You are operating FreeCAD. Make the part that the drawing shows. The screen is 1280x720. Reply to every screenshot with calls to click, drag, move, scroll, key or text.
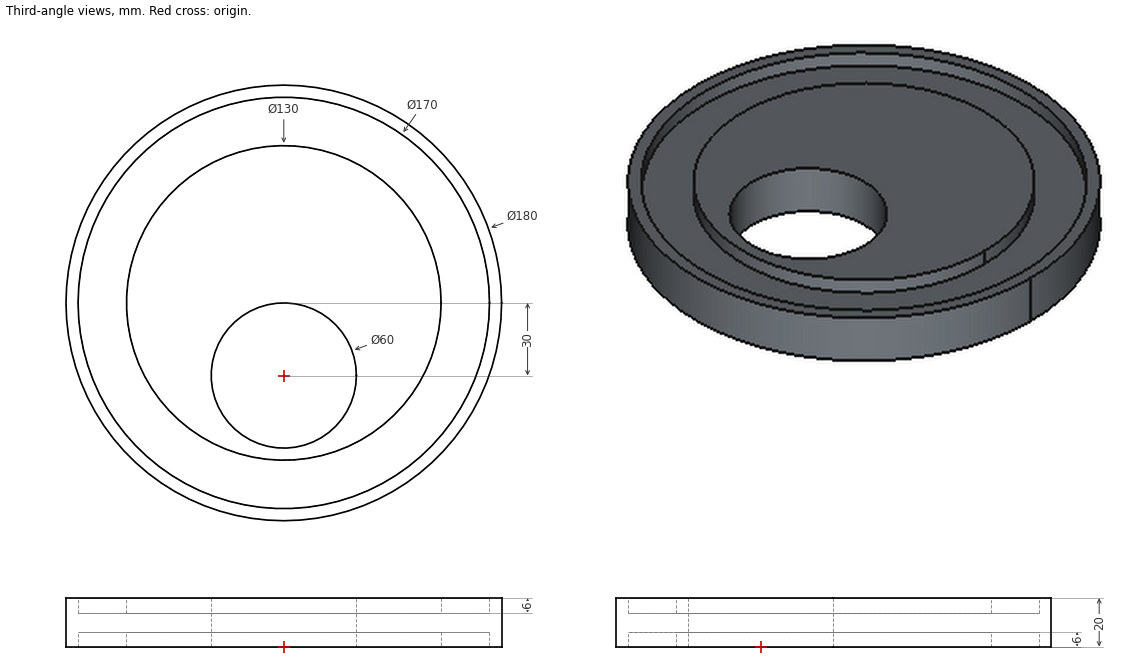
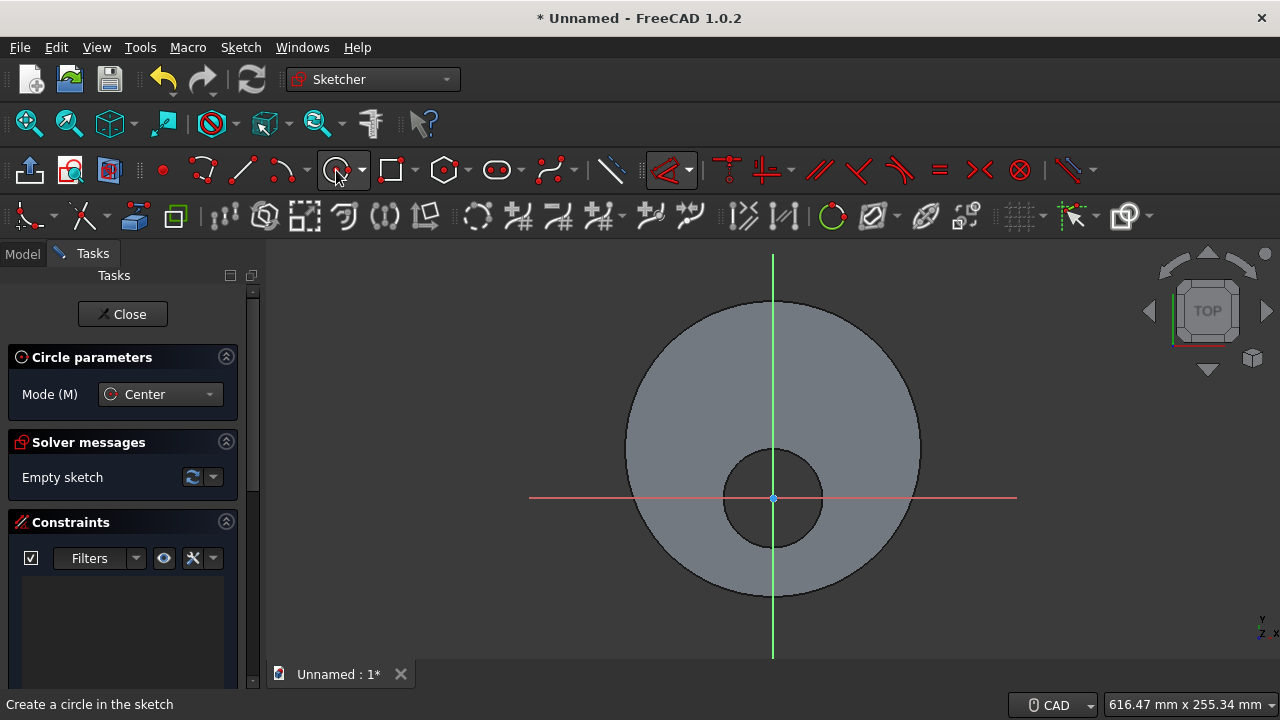
click(773, 449)
move(872, 350)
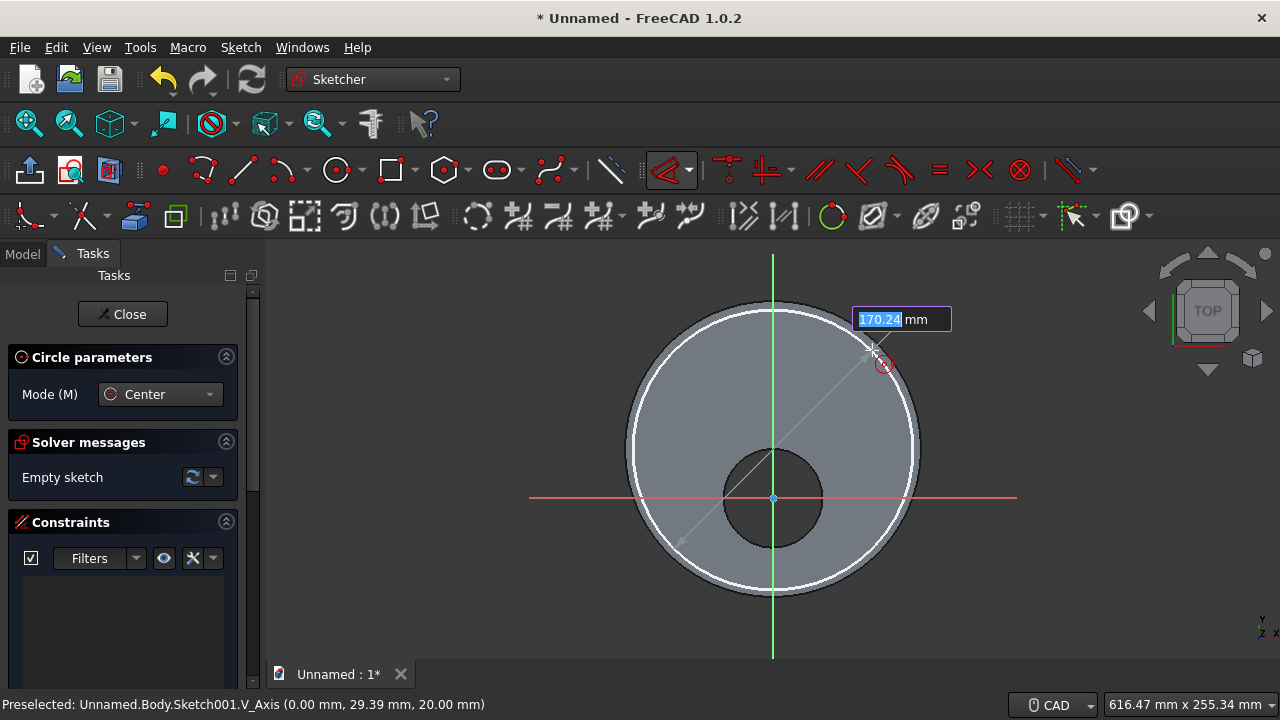
text(170)
key(Return)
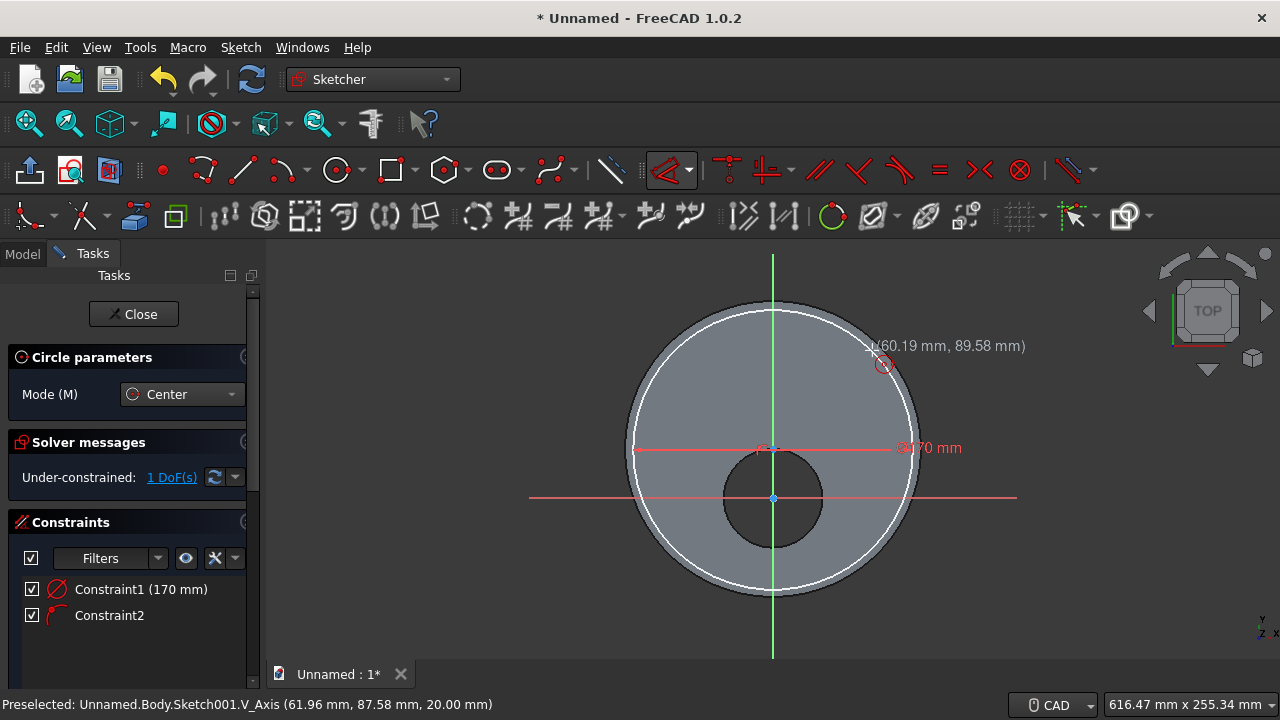
click(773, 450)
move(849, 373)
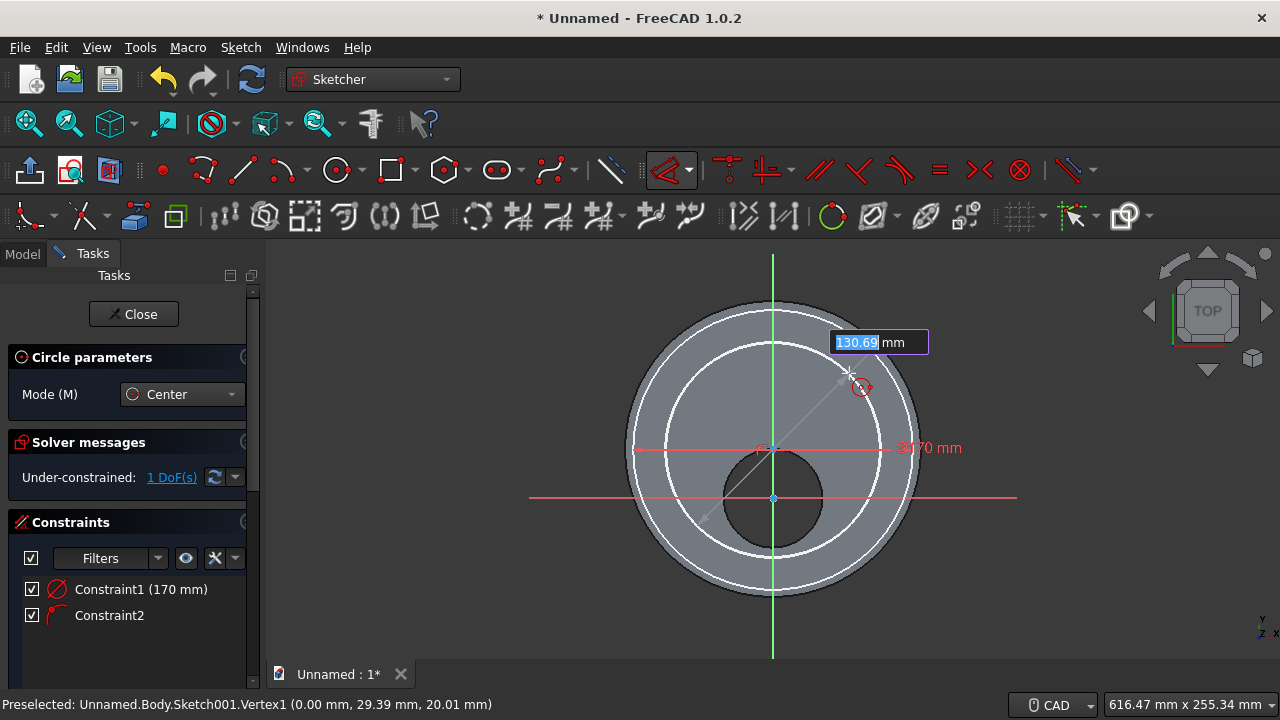
text(130)
key(Return)
key(Escape)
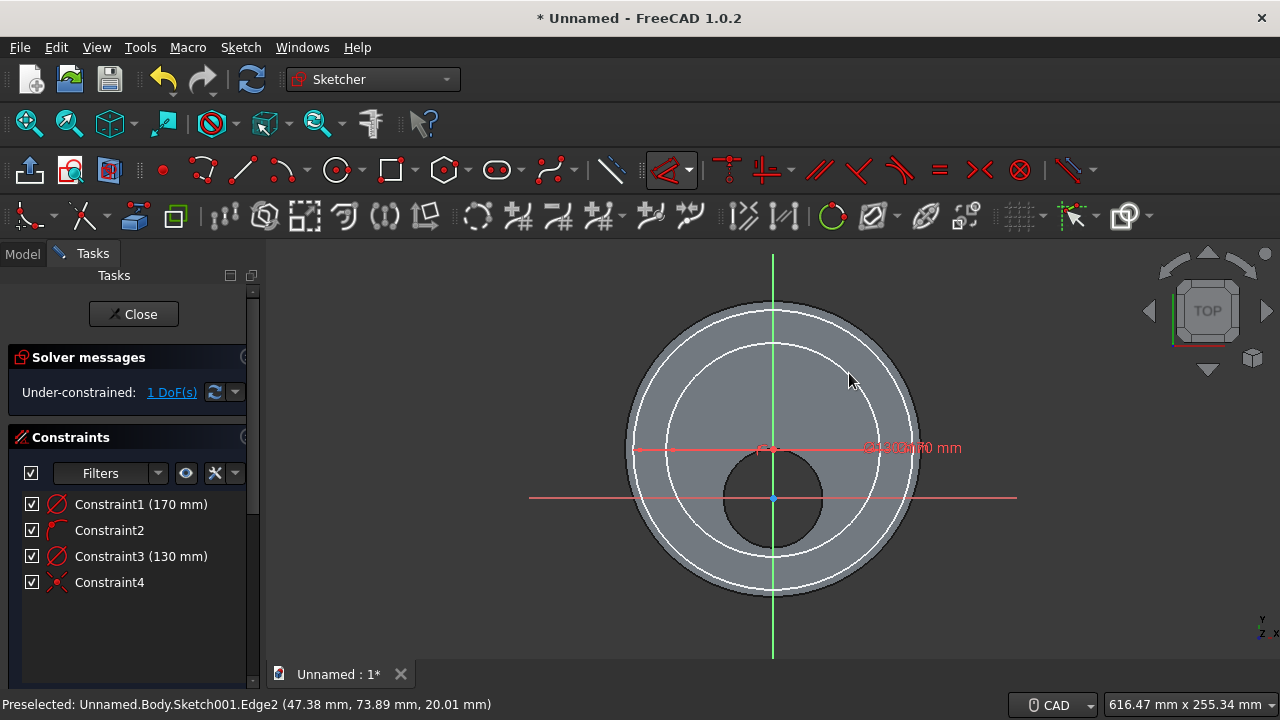
click(773, 450)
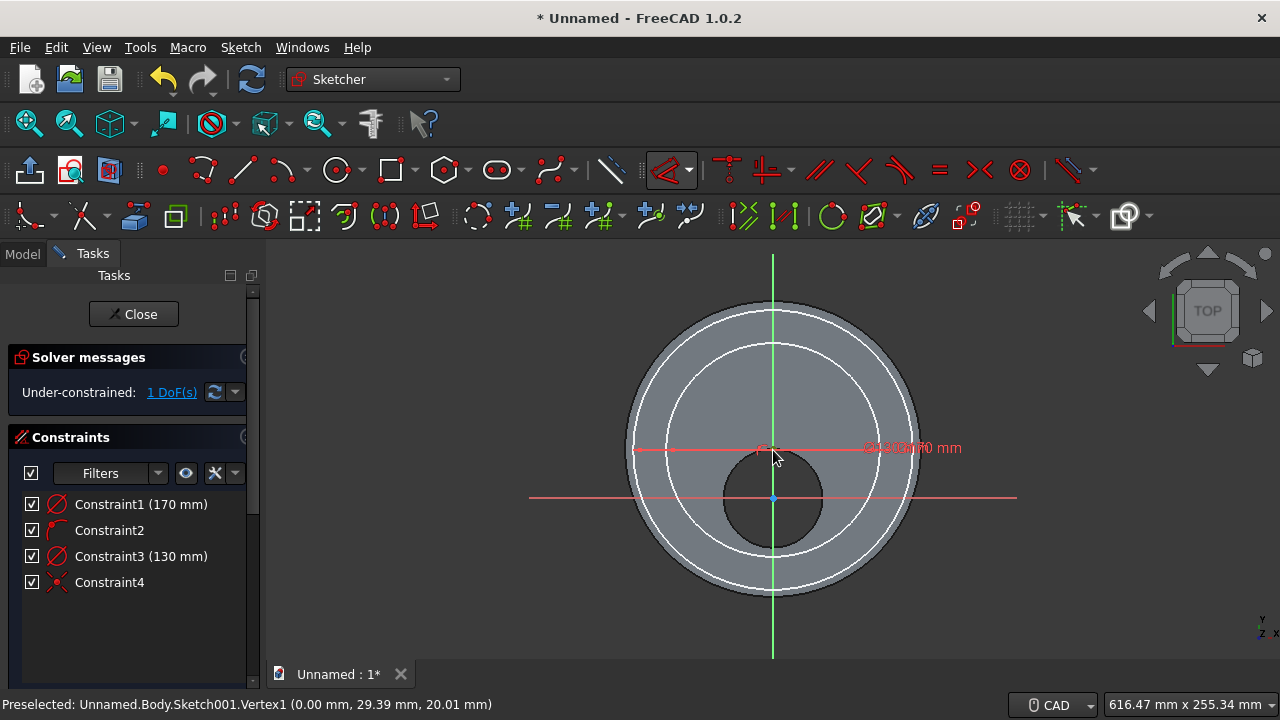
click(692, 170)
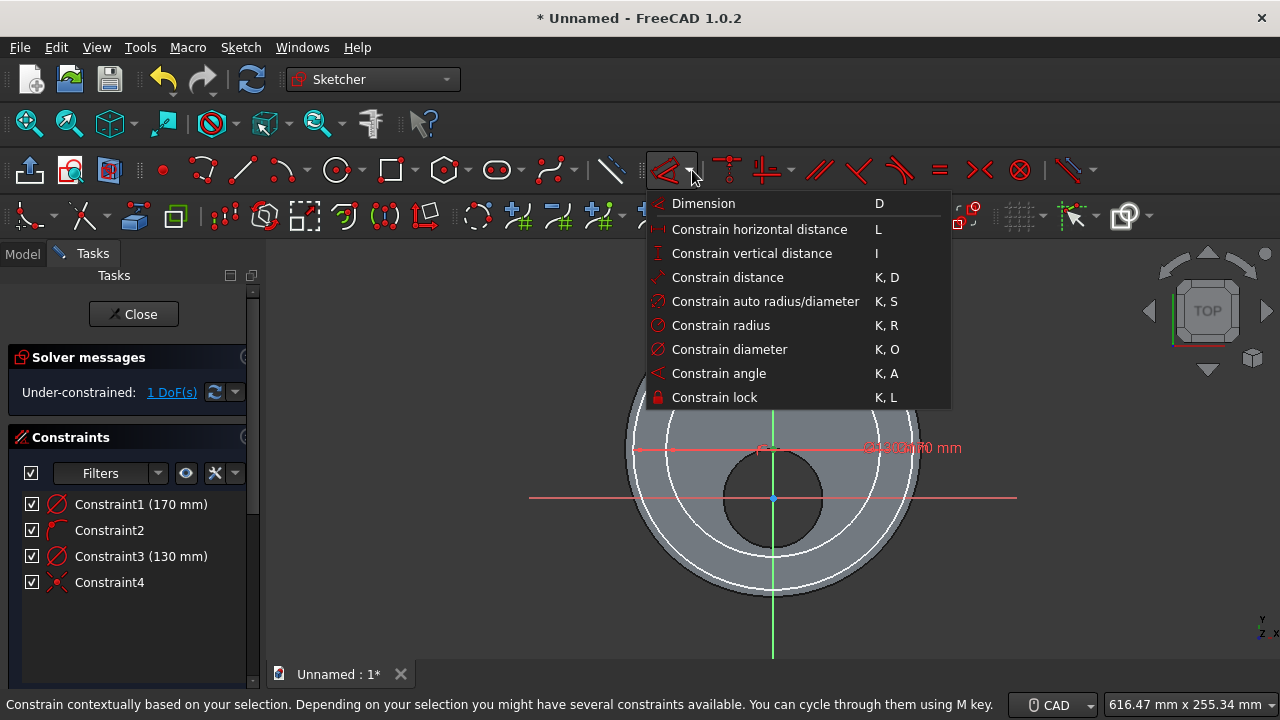
click(799, 253)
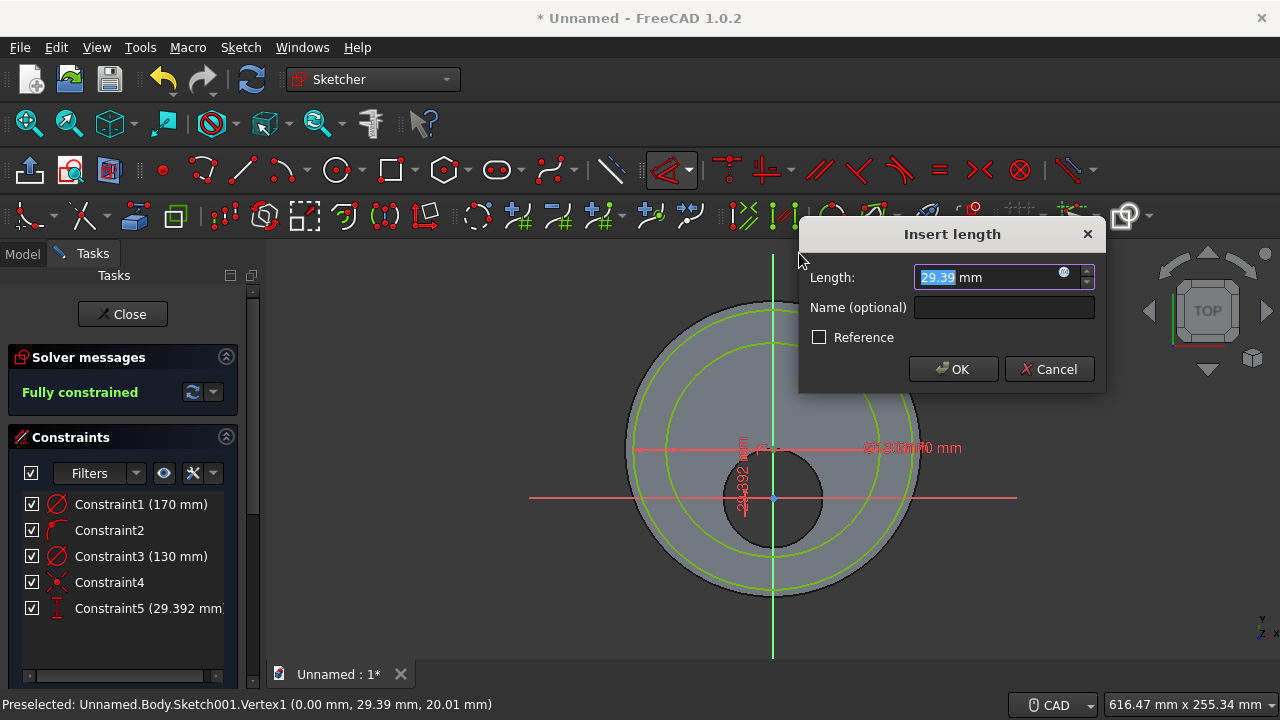
text(30)
key(Return)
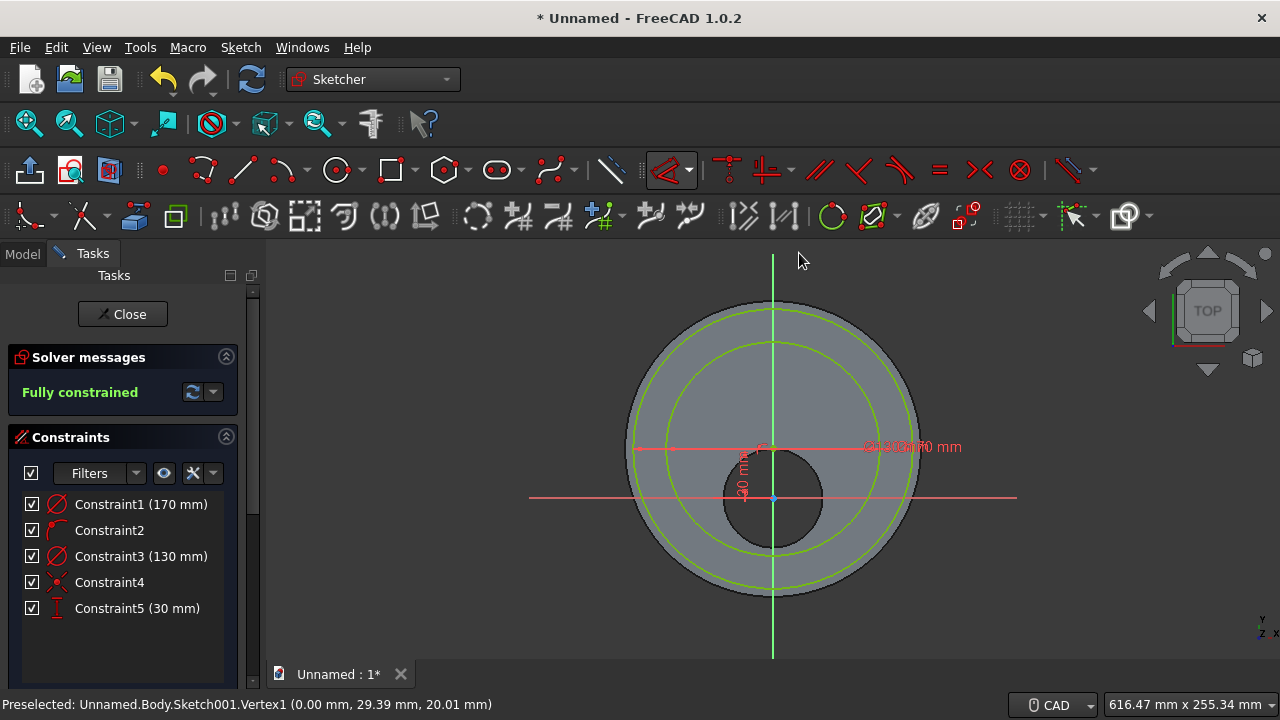
click(123, 314)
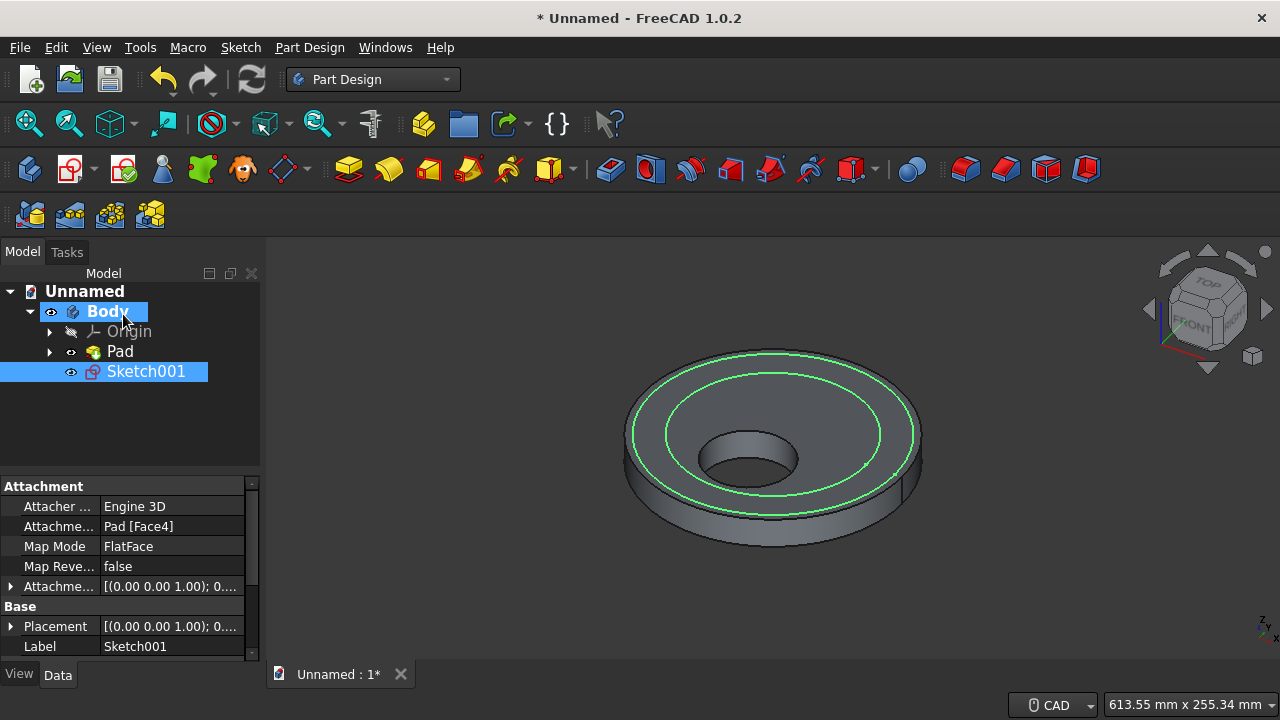
click(612, 170)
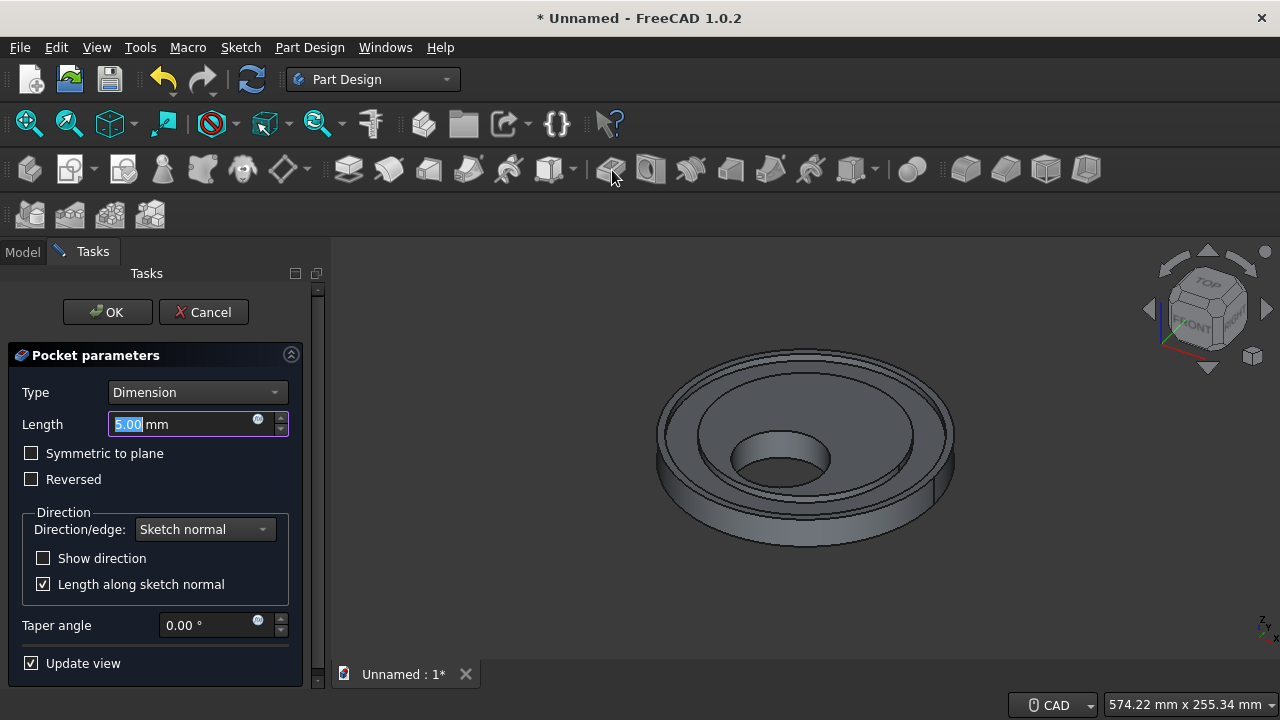
text(6)
key(Tab)